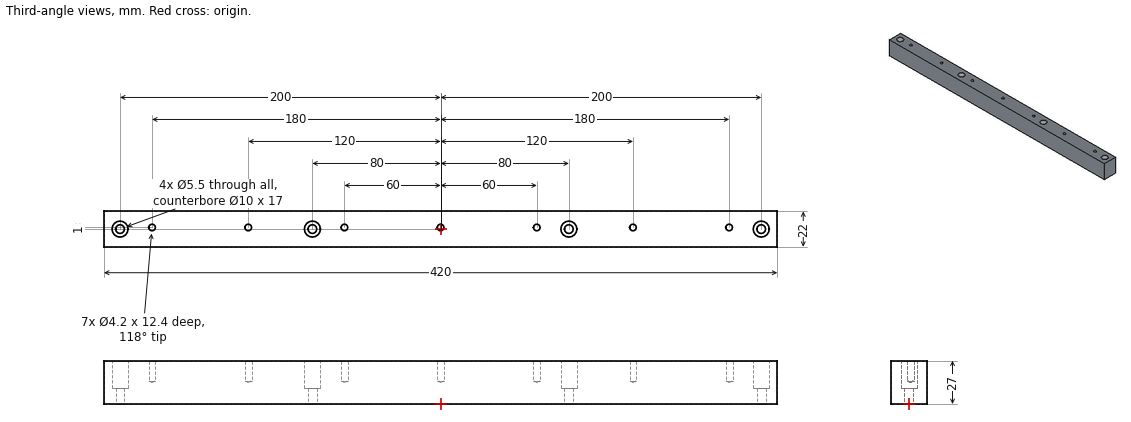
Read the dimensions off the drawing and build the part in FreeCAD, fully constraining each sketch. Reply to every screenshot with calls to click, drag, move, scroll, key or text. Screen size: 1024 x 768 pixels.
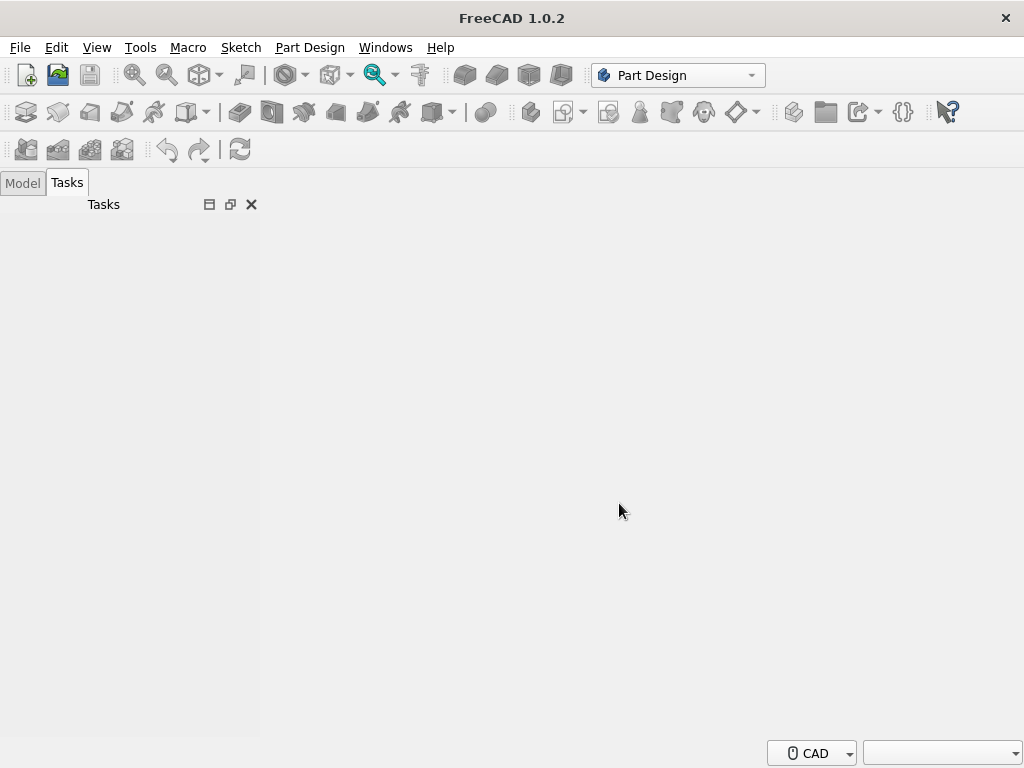
click(26, 76)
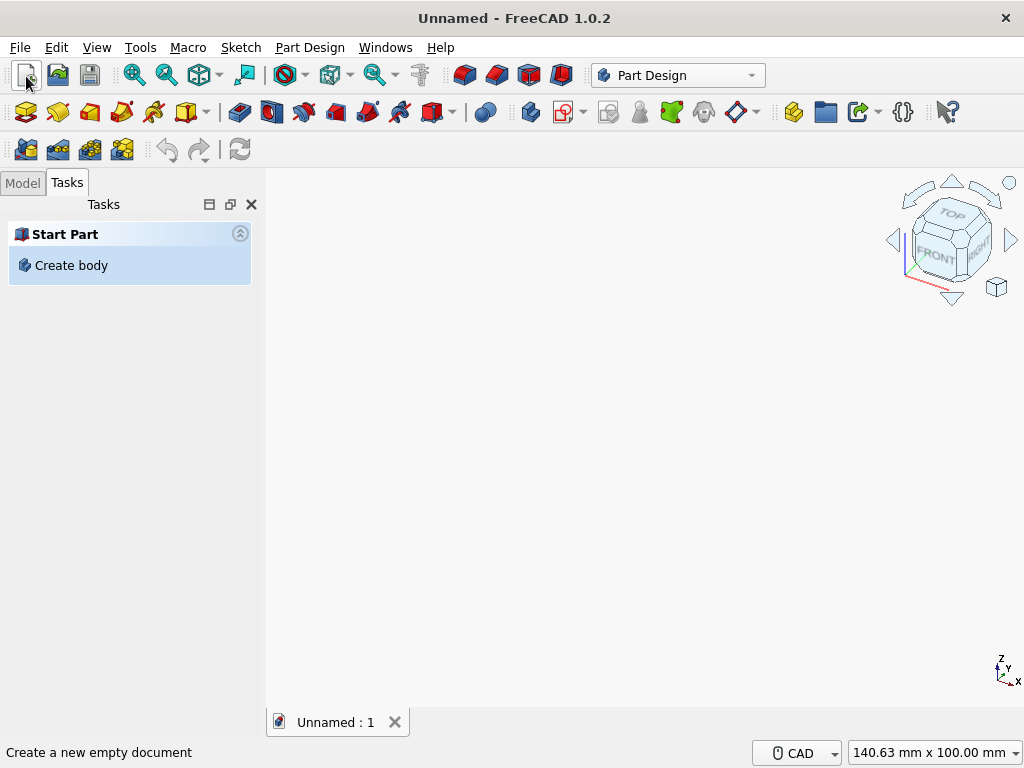
click(564, 112)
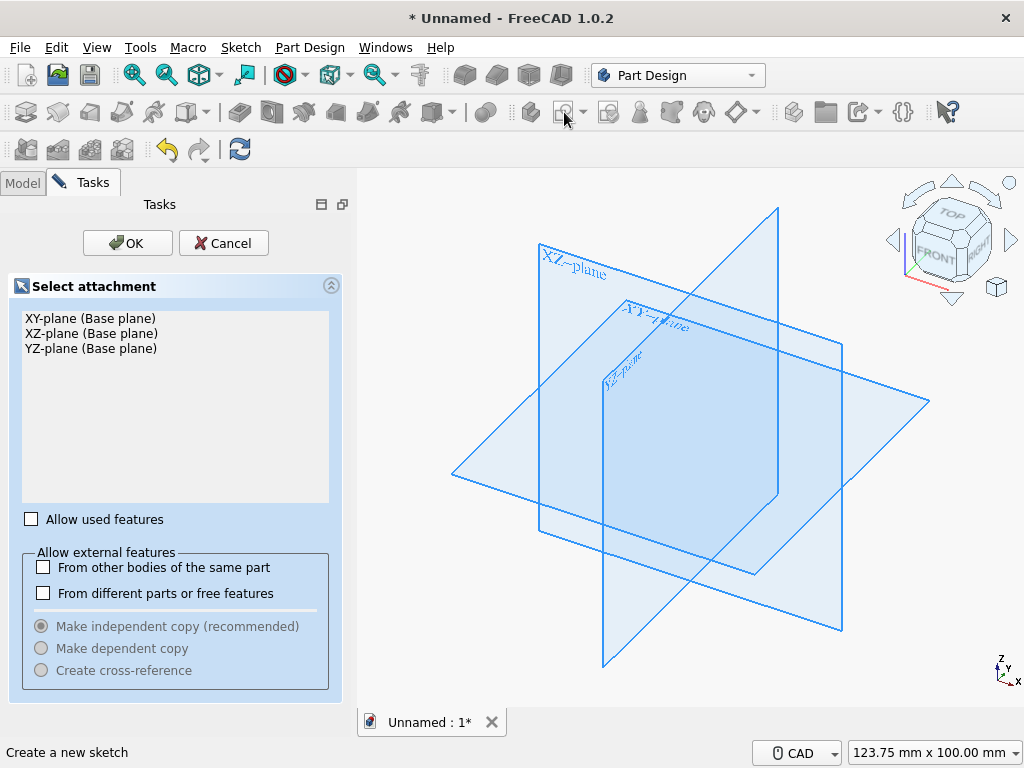
click(82, 318)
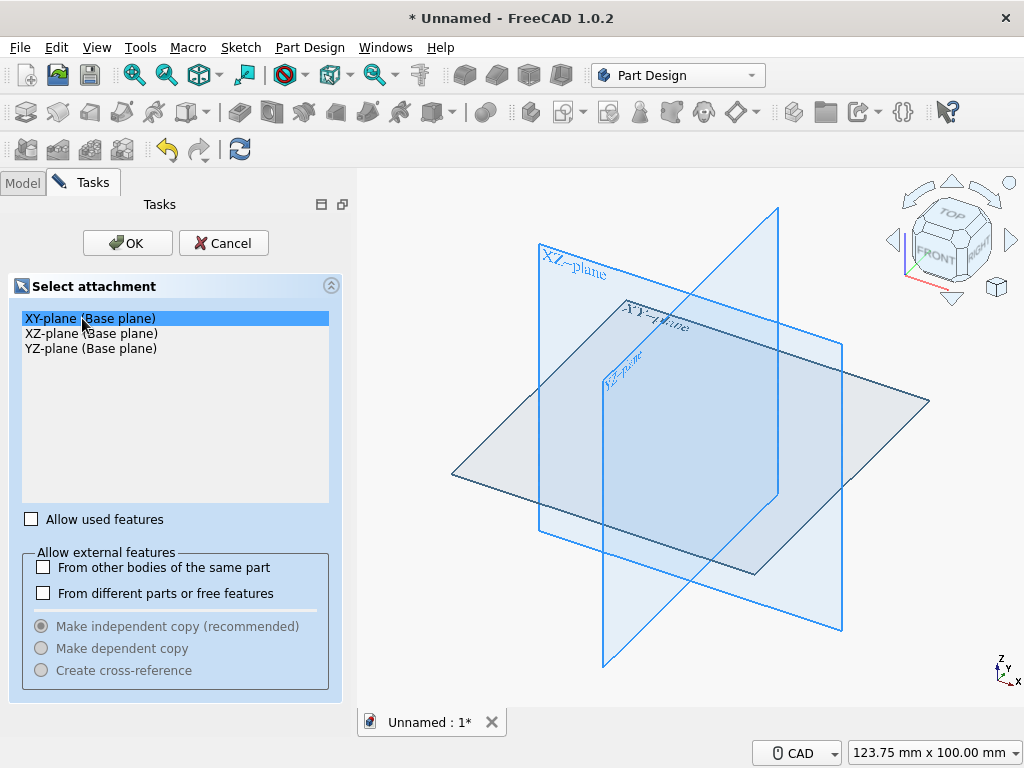
click(128, 243)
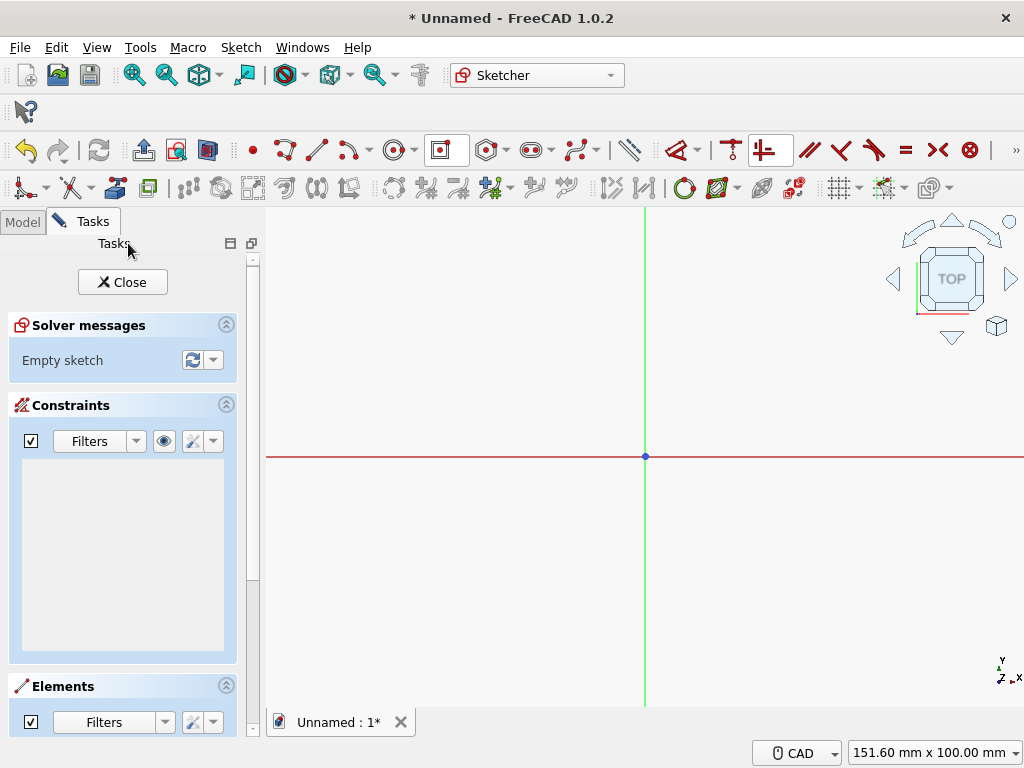
scroll(559, 457, down, 8)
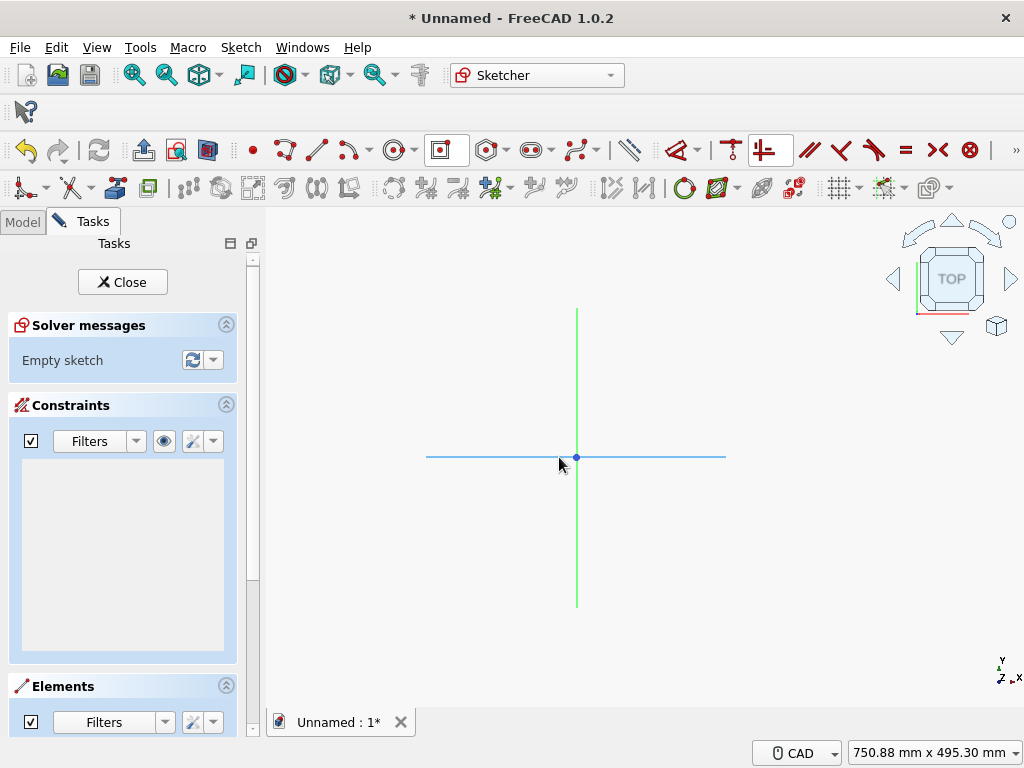
key(g)
key(v)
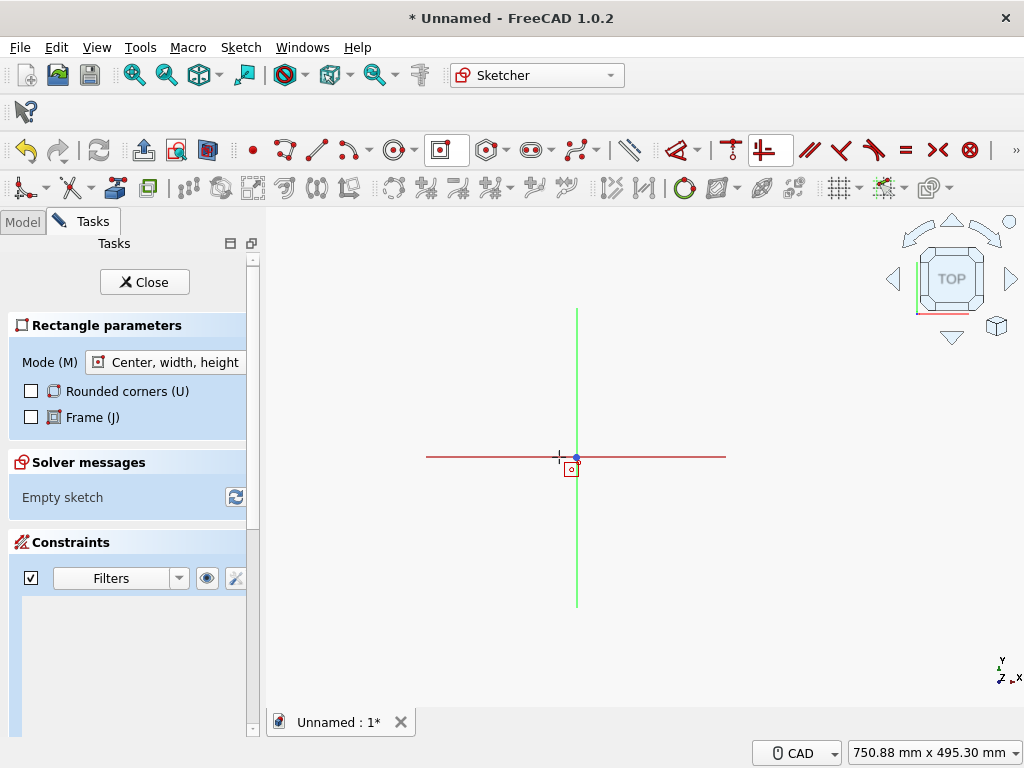
scroll(577, 457, up, 2)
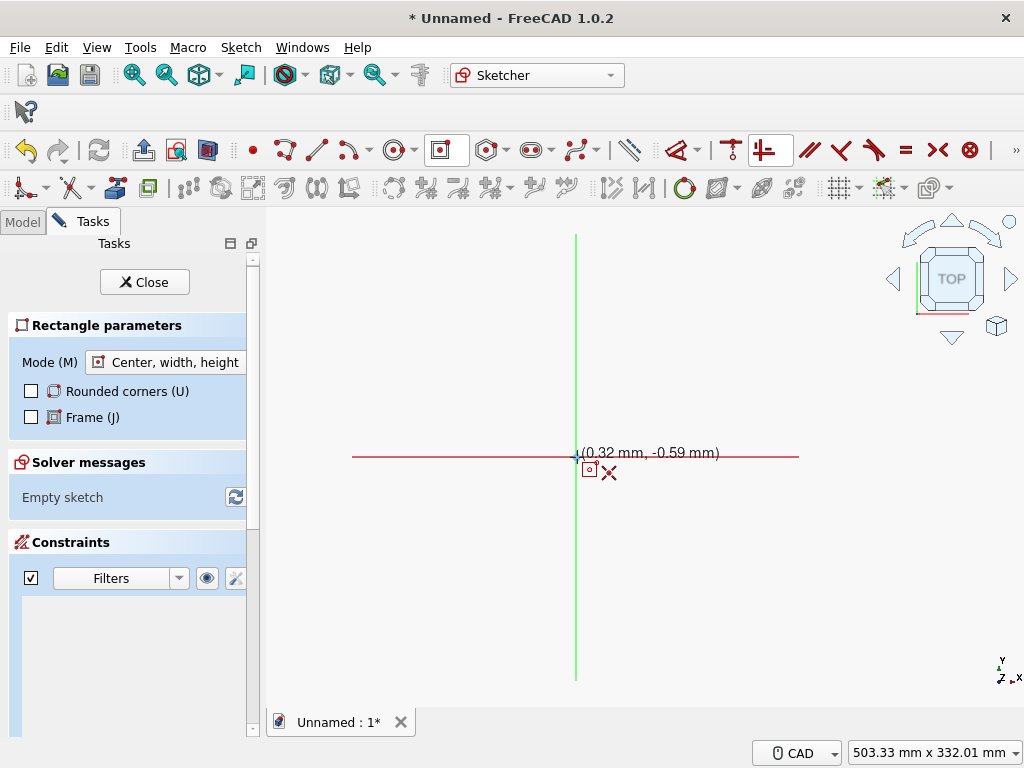
click(576, 457)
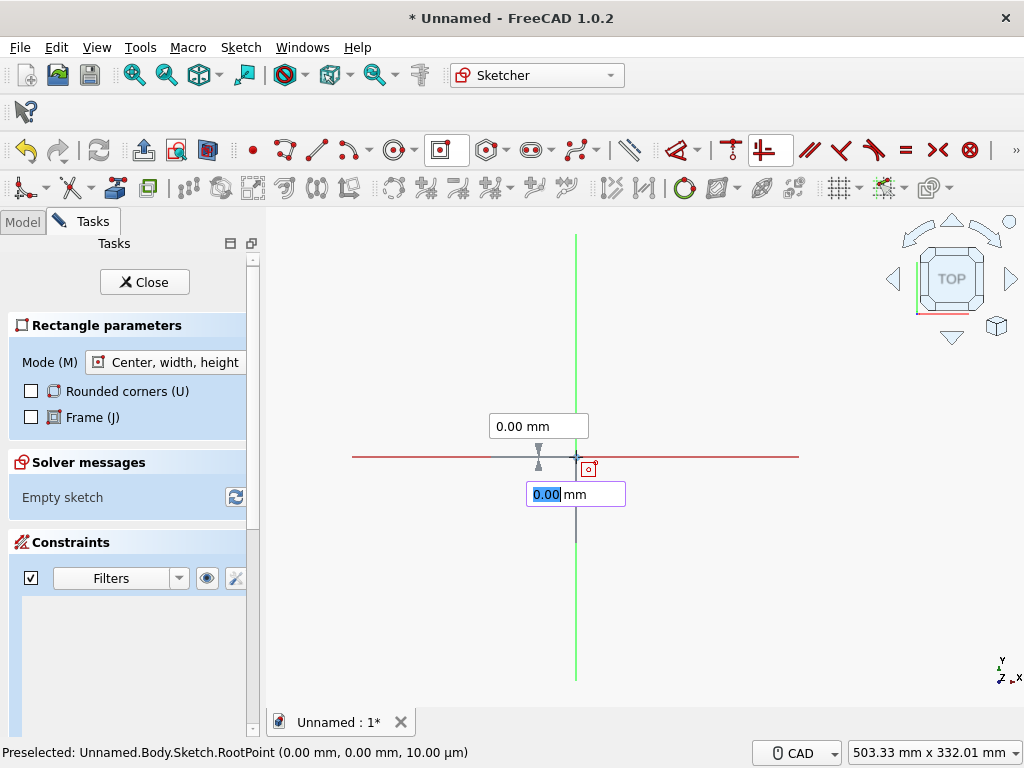
scroll(577, 456, down, 2)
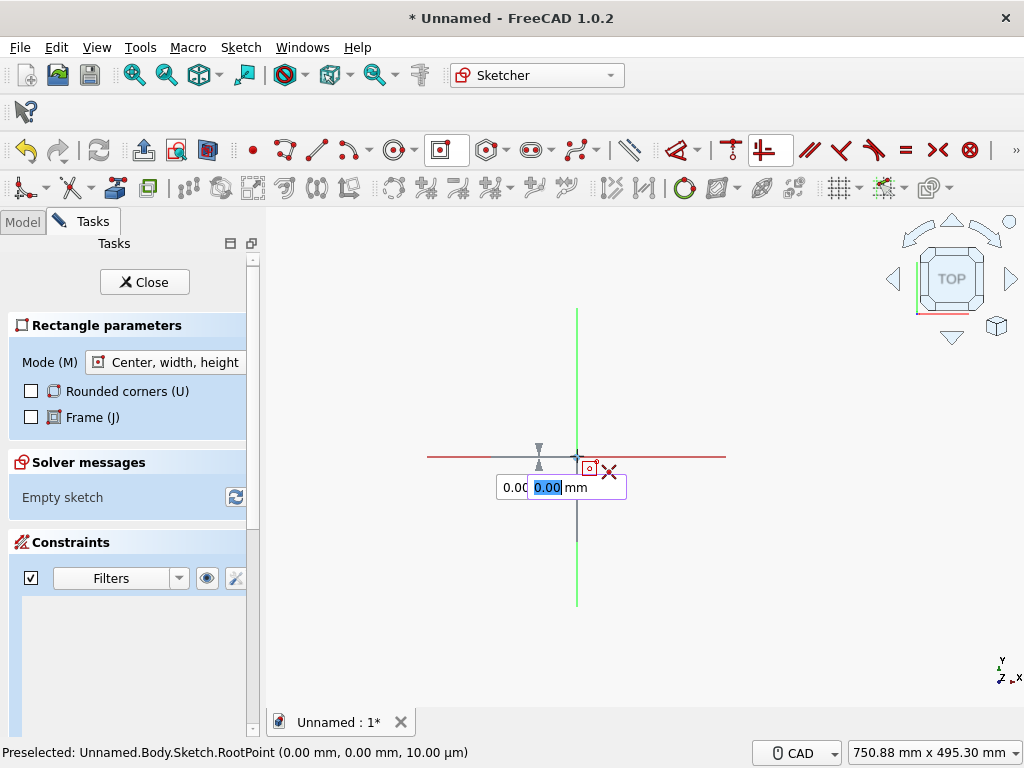
scroll(789, 446, up, 2)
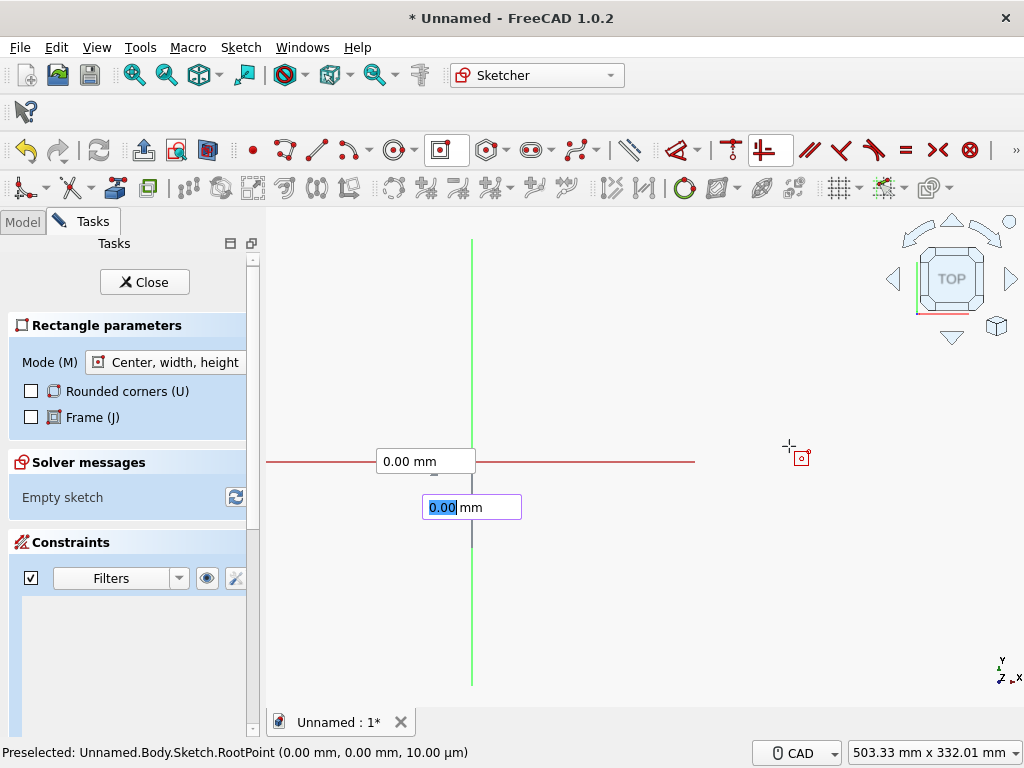
click(788, 446)
key(Escape)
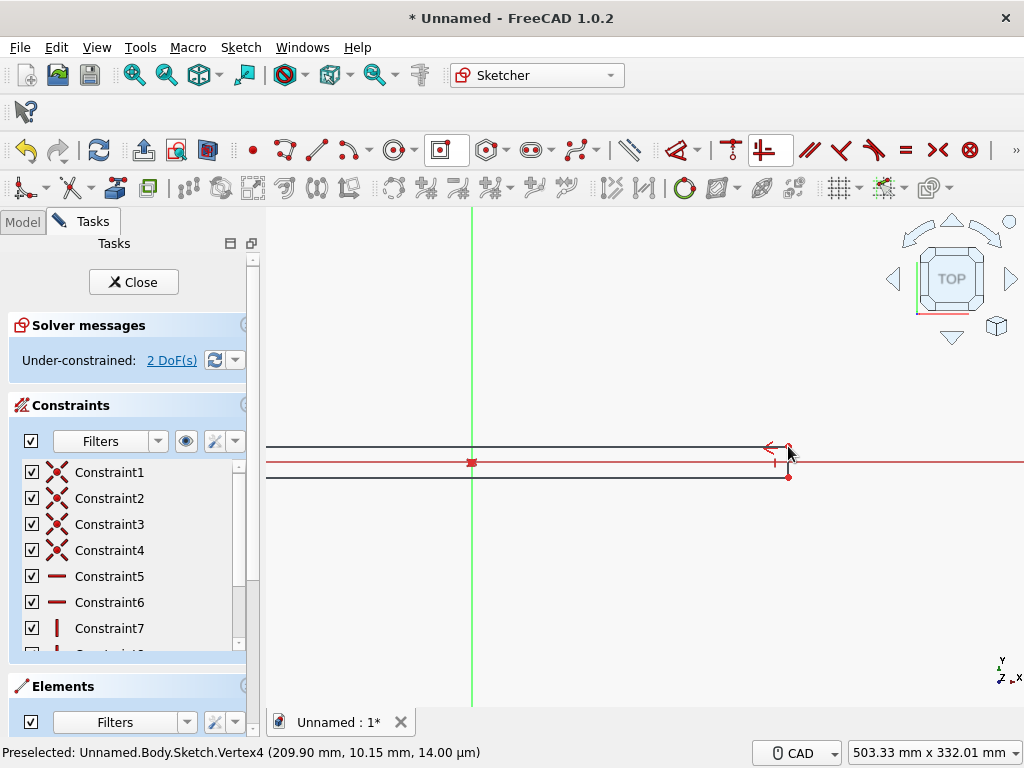
key(d)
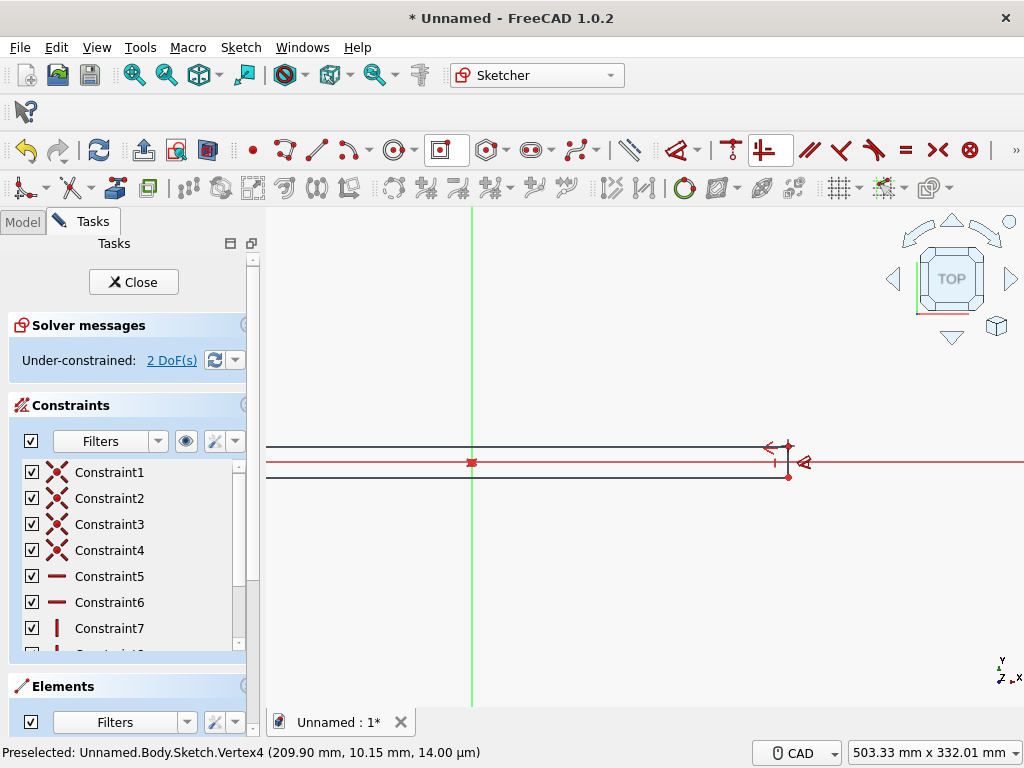
click(788, 465)
click(822, 455)